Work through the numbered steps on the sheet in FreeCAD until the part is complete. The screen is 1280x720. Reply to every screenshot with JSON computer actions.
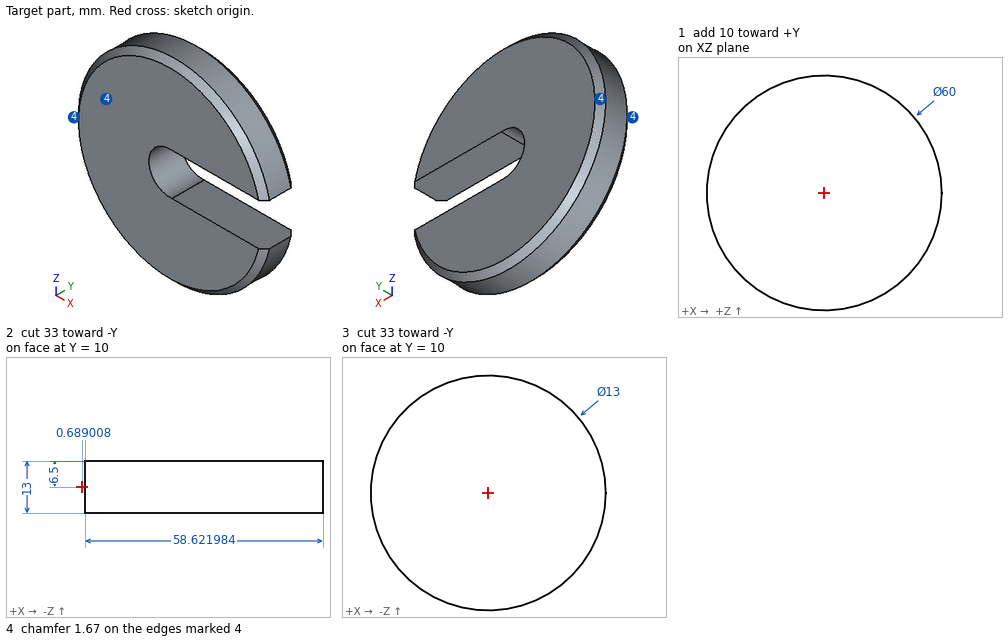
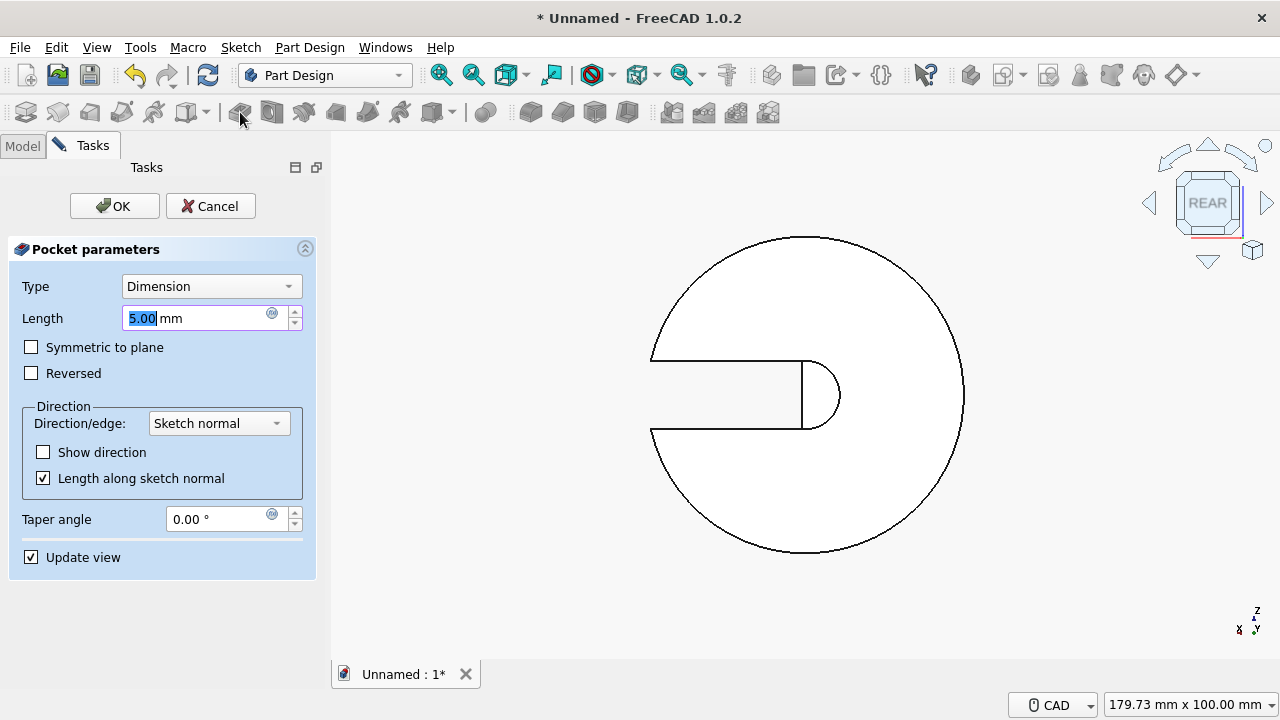
{"action": "type", "text": "33"}
{"action": "key", "text": "Tab"}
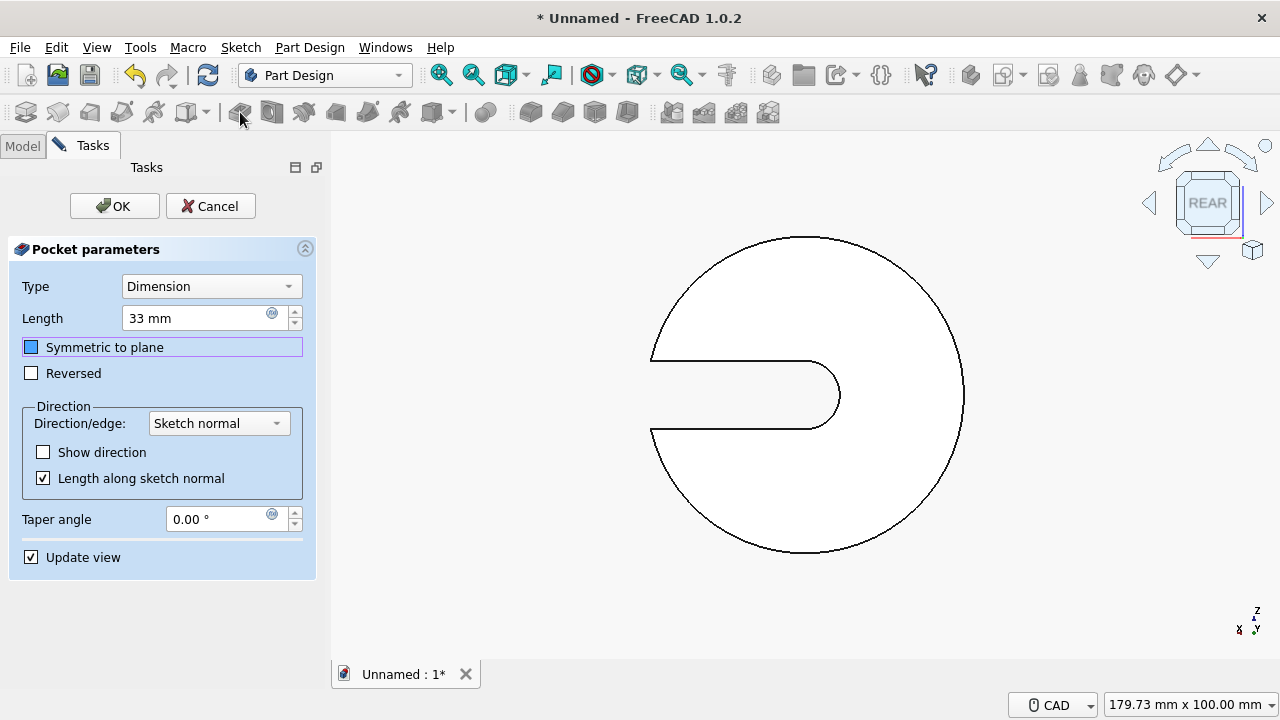
{"action": "left_click", "coordinate": [115, 206]}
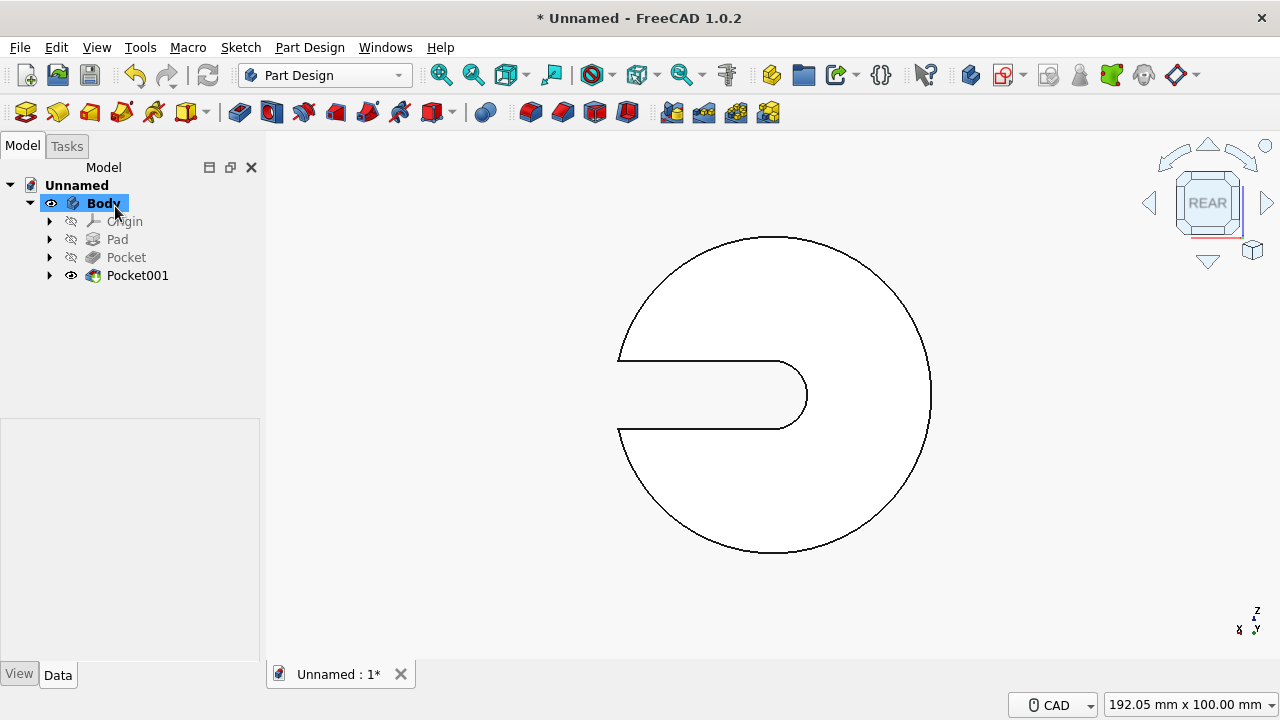
{"action": "left_click", "coordinate": [931, 394]}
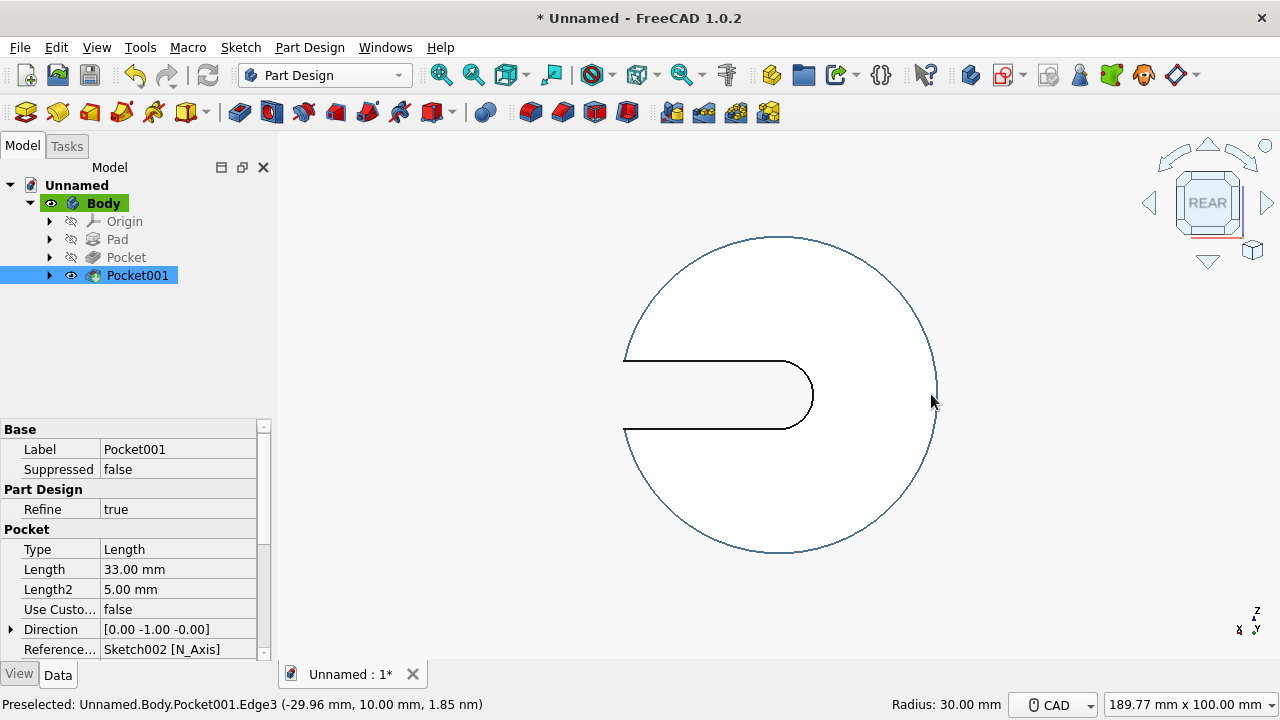
{"action": "key", "text": "0"}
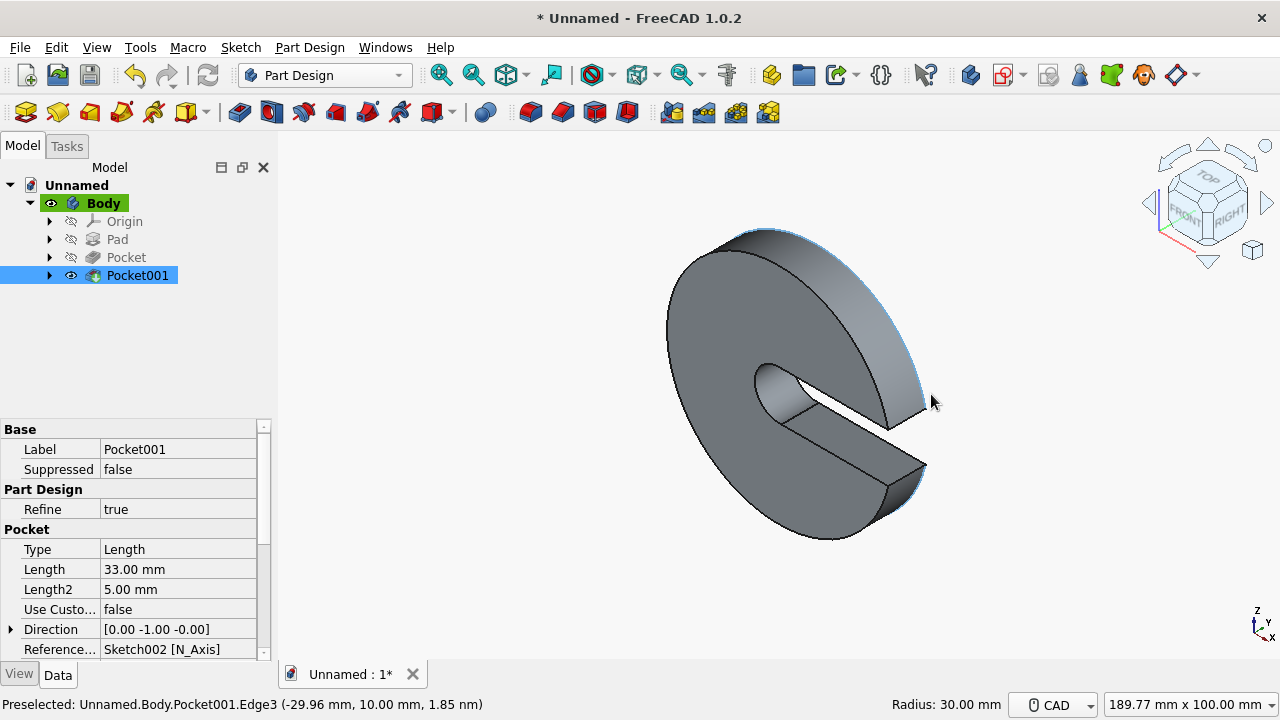
{"action": "left_click", "coordinate": [735, 250], "text": "ctrl"}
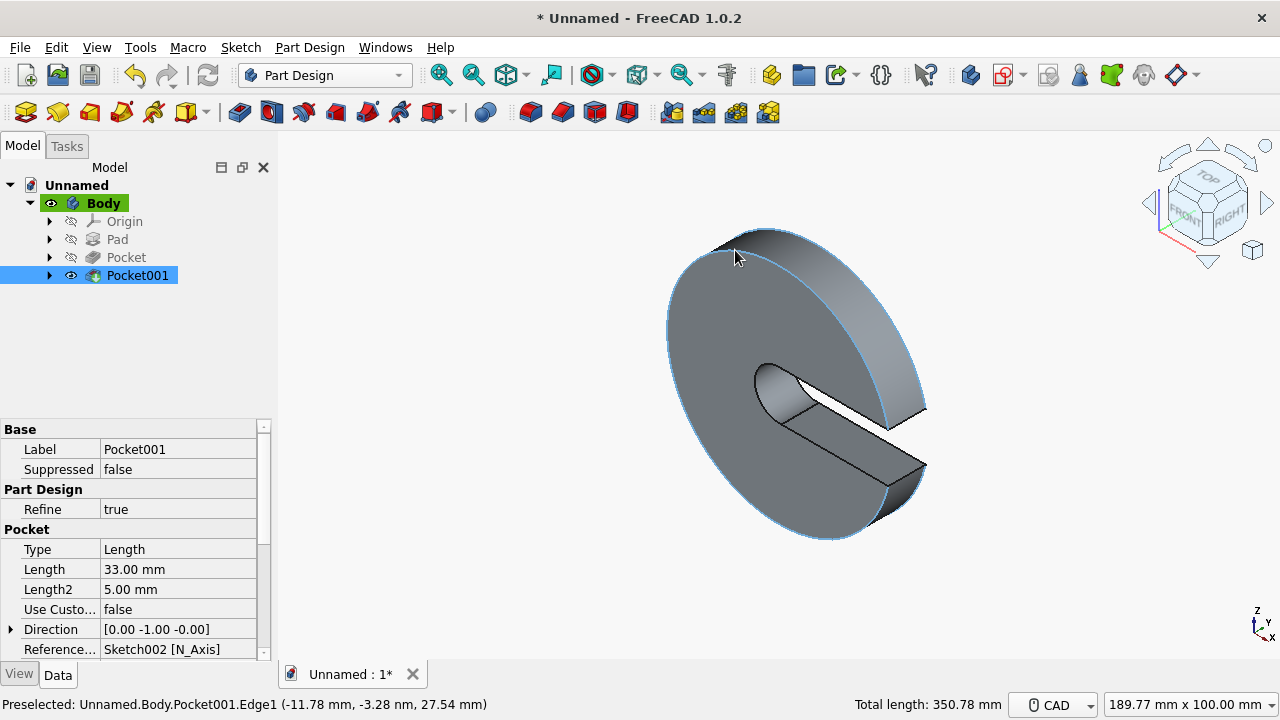
{"action": "left_click", "coordinate": [564, 112]}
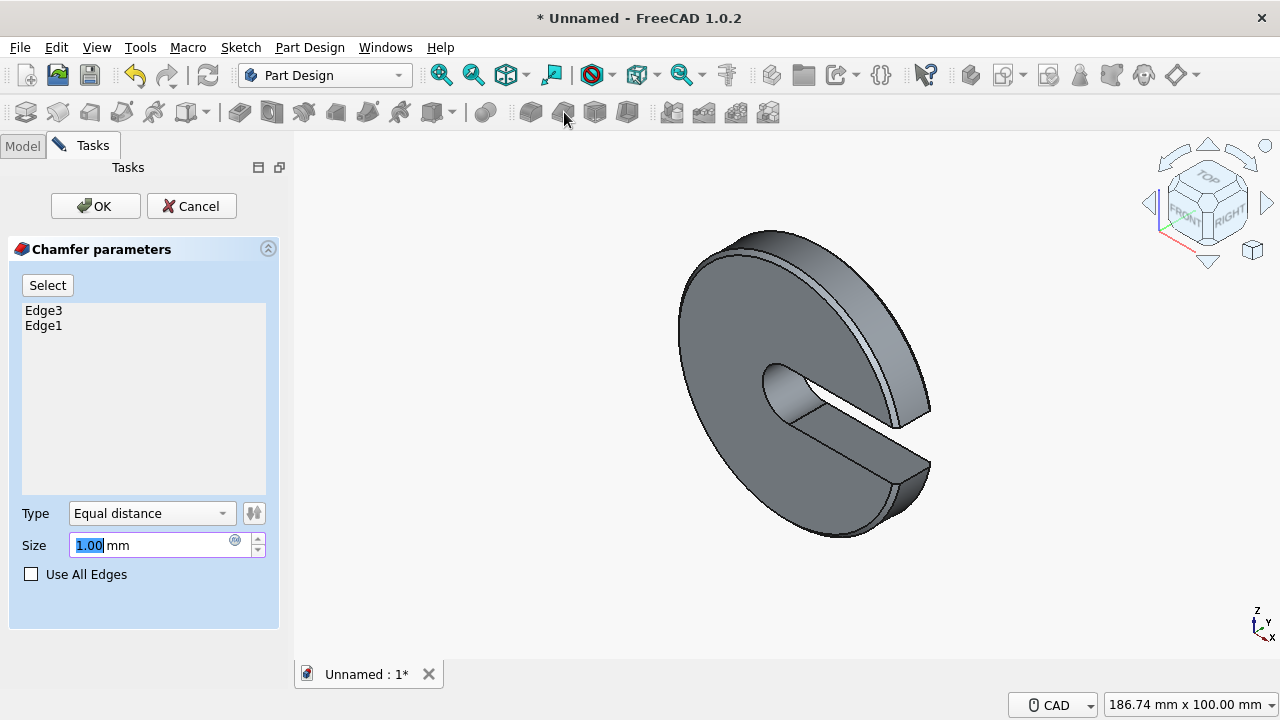
{"action": "type", "text": "1.67"}
{"action": "key", "text": "Tab"}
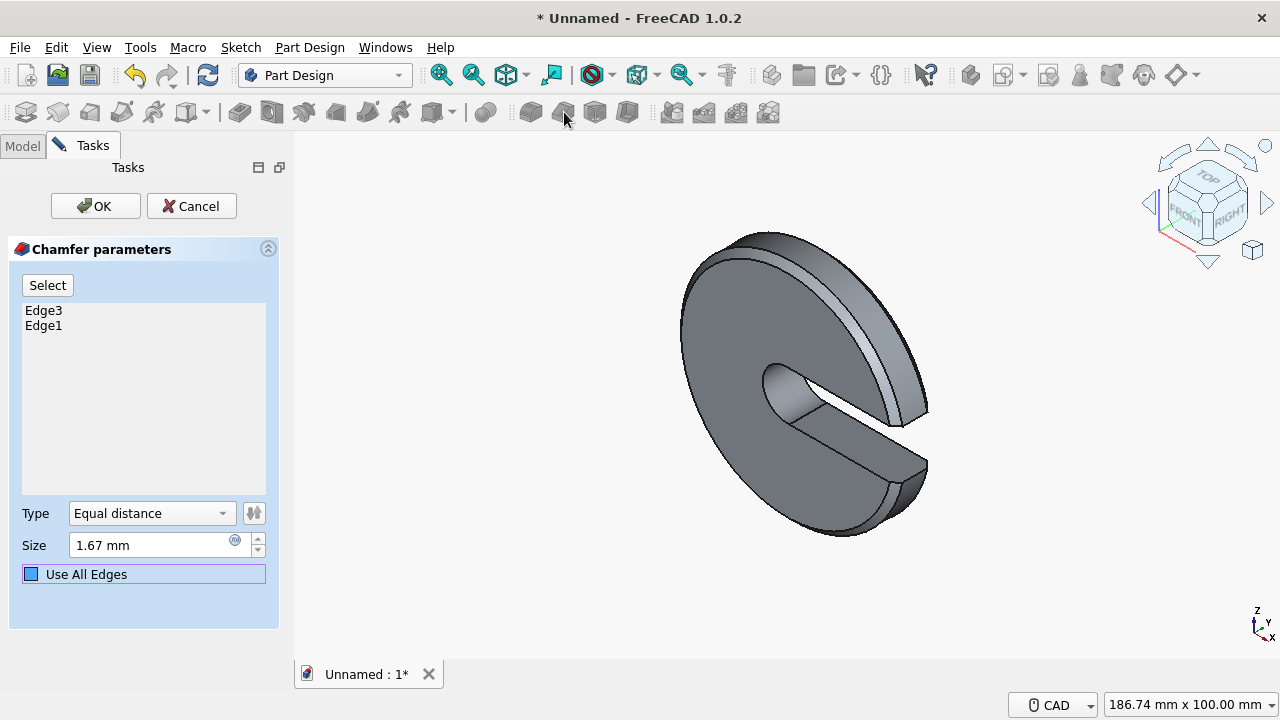
{"action": "left_click", "coordinate": [96, 206]}